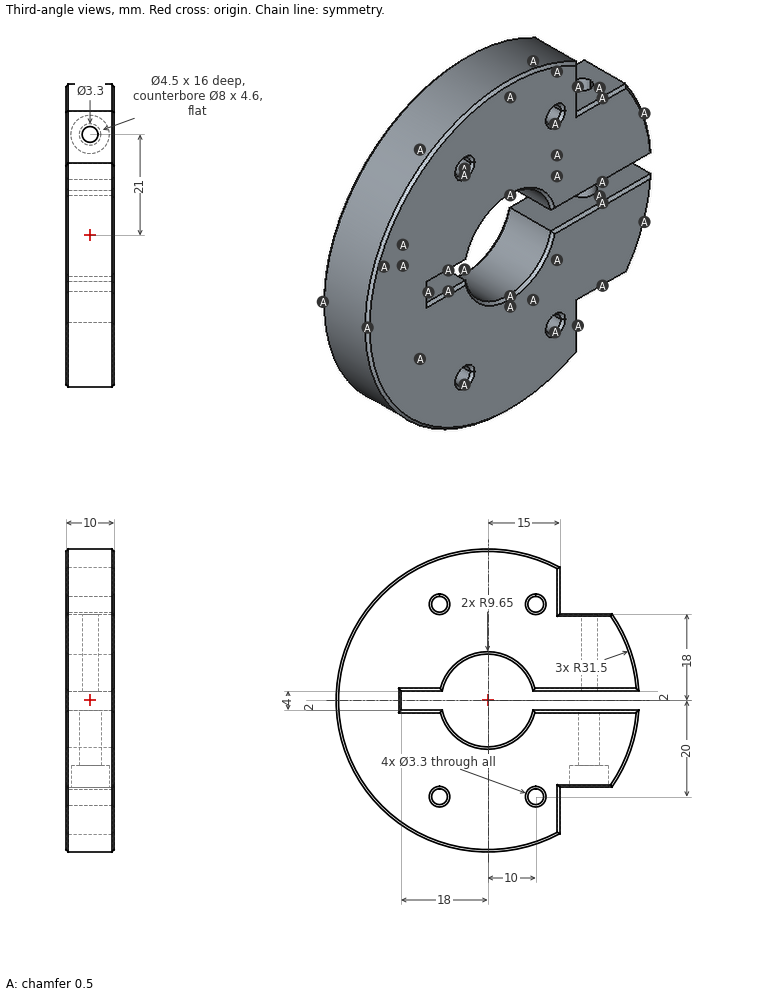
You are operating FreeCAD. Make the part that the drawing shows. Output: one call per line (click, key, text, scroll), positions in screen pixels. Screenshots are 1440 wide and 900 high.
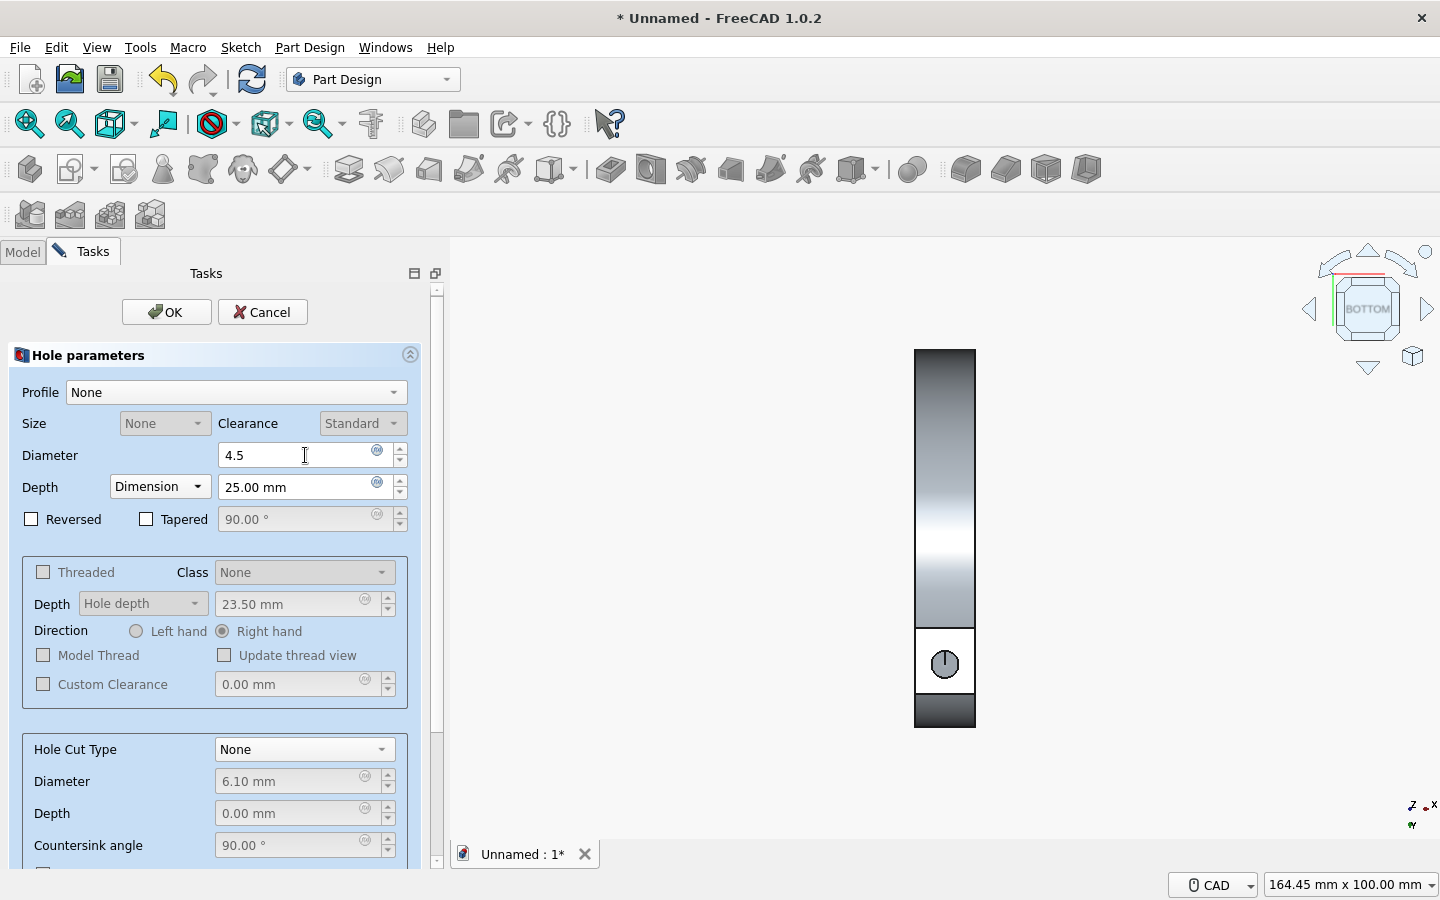
triple_click(305, 487)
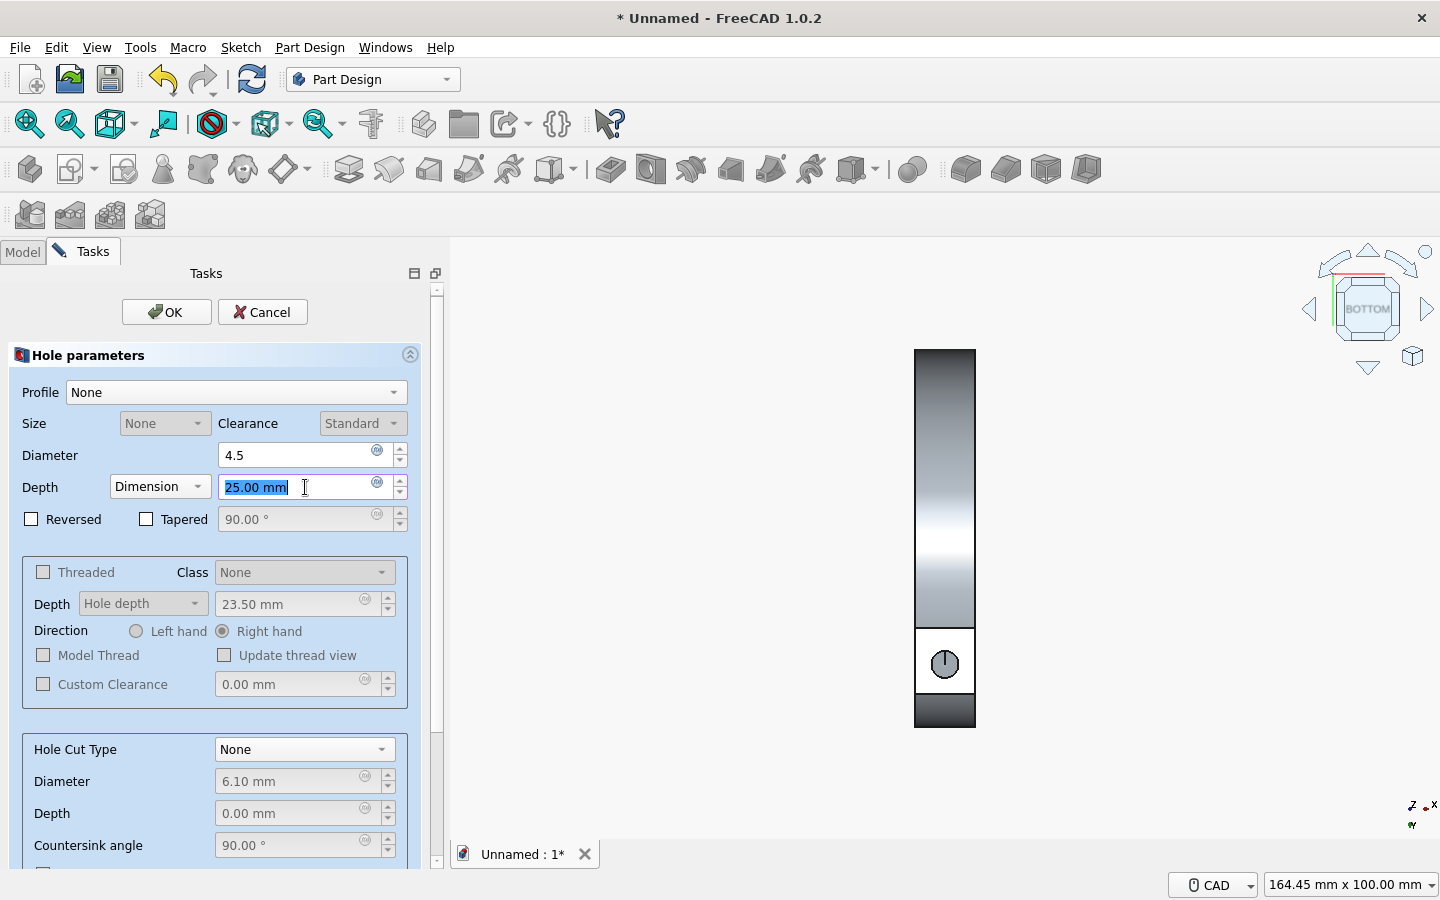
text(16)
key(Tab)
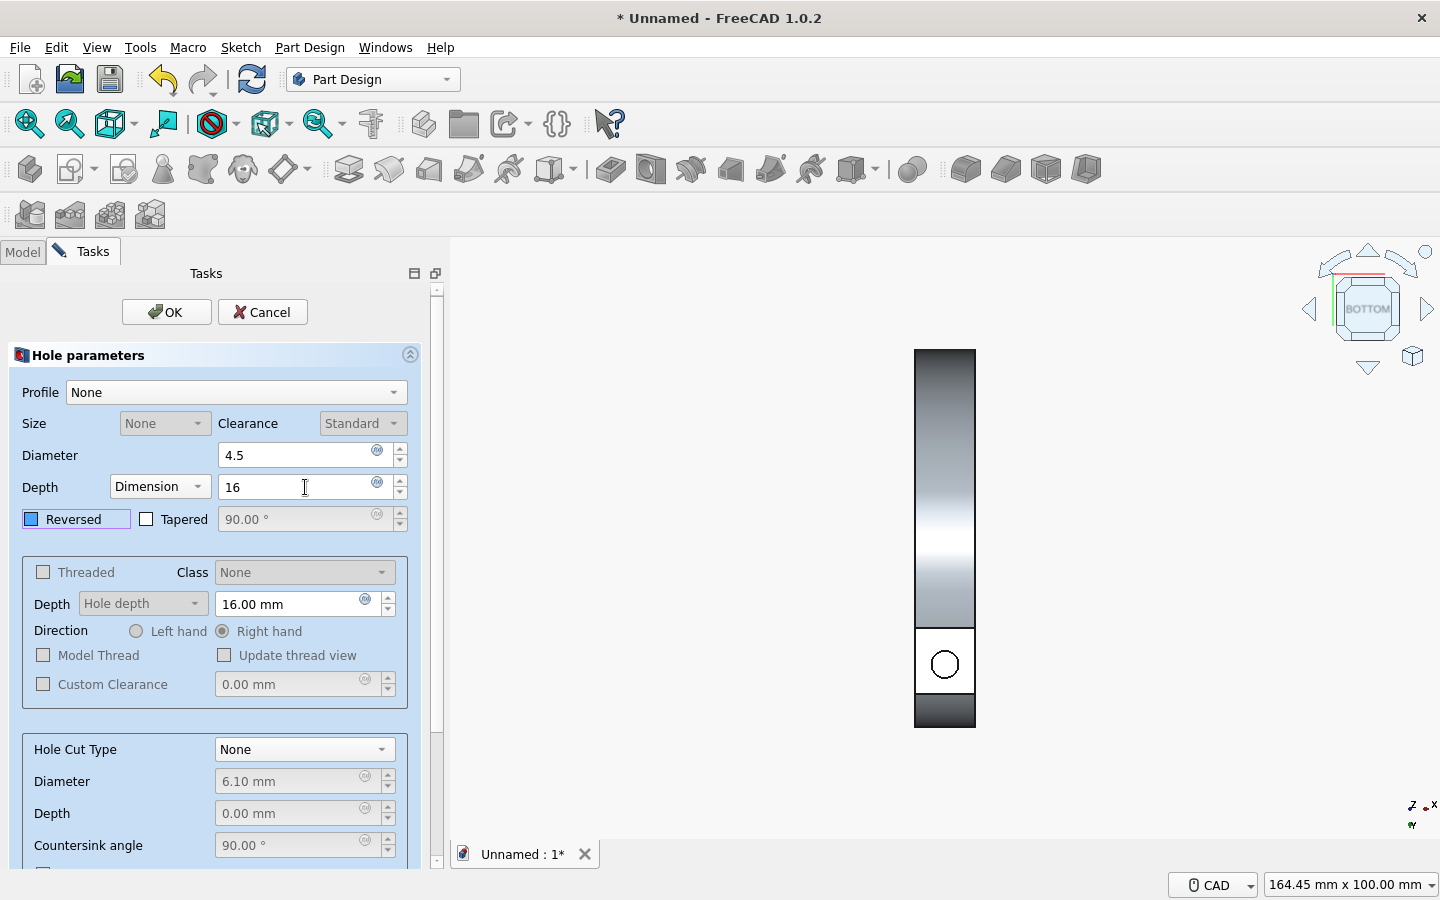
click(306, 750)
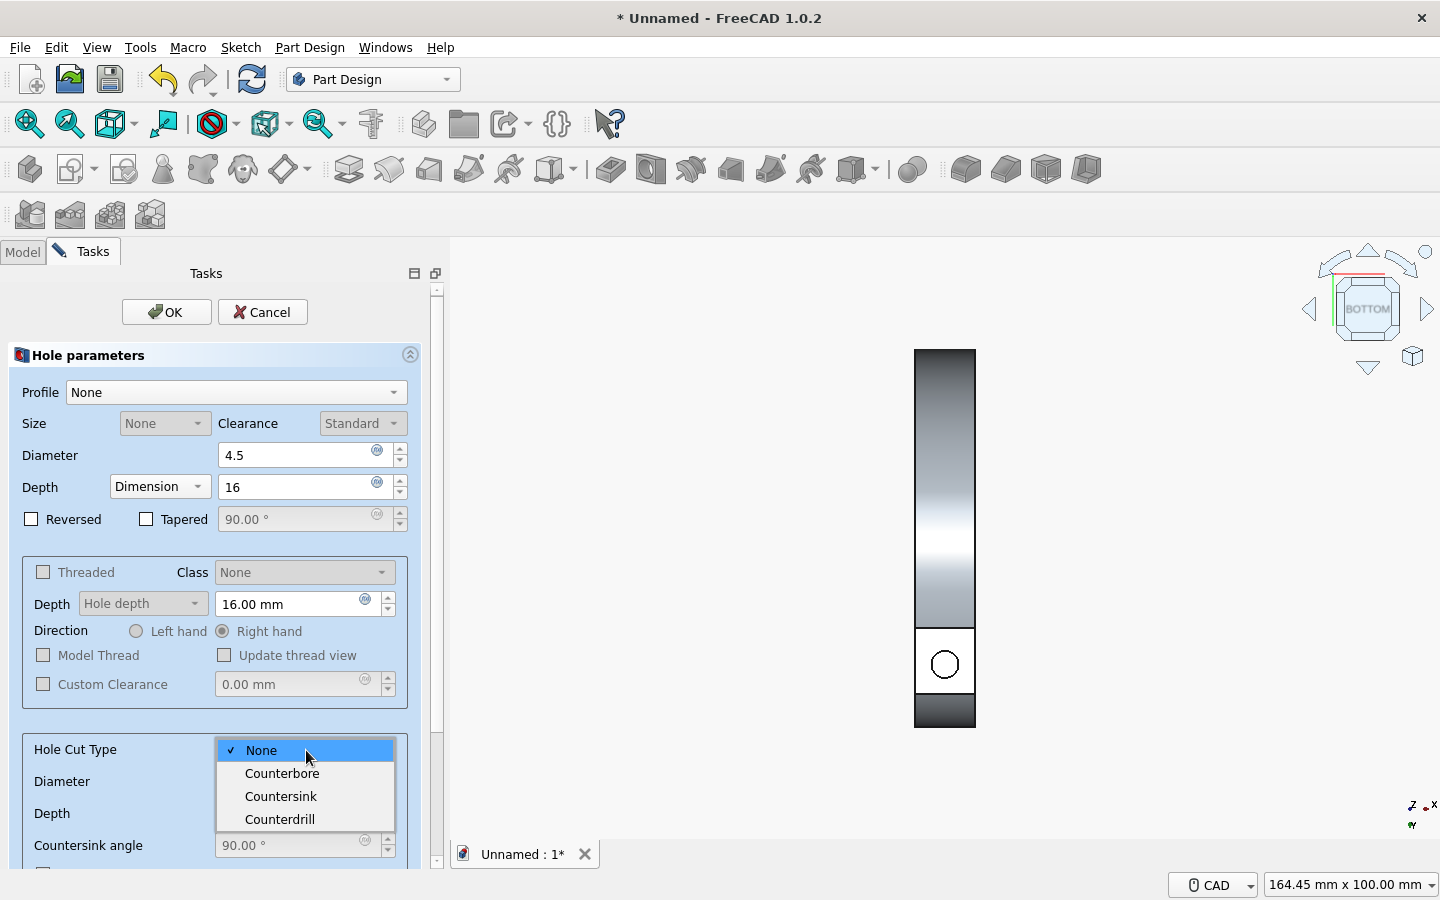
click(304, 774)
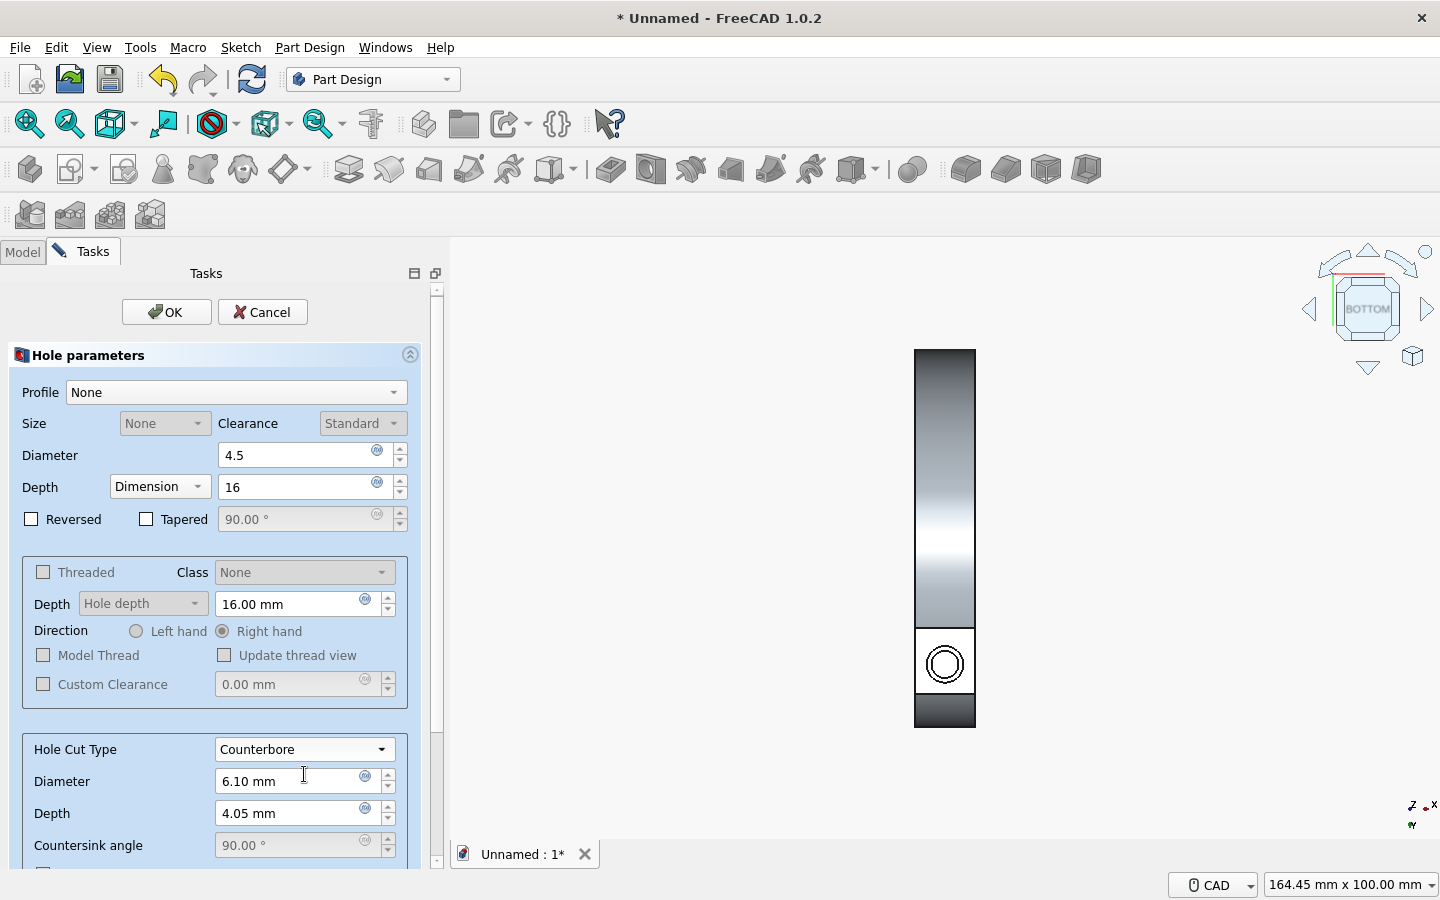
triple_click(298, 781)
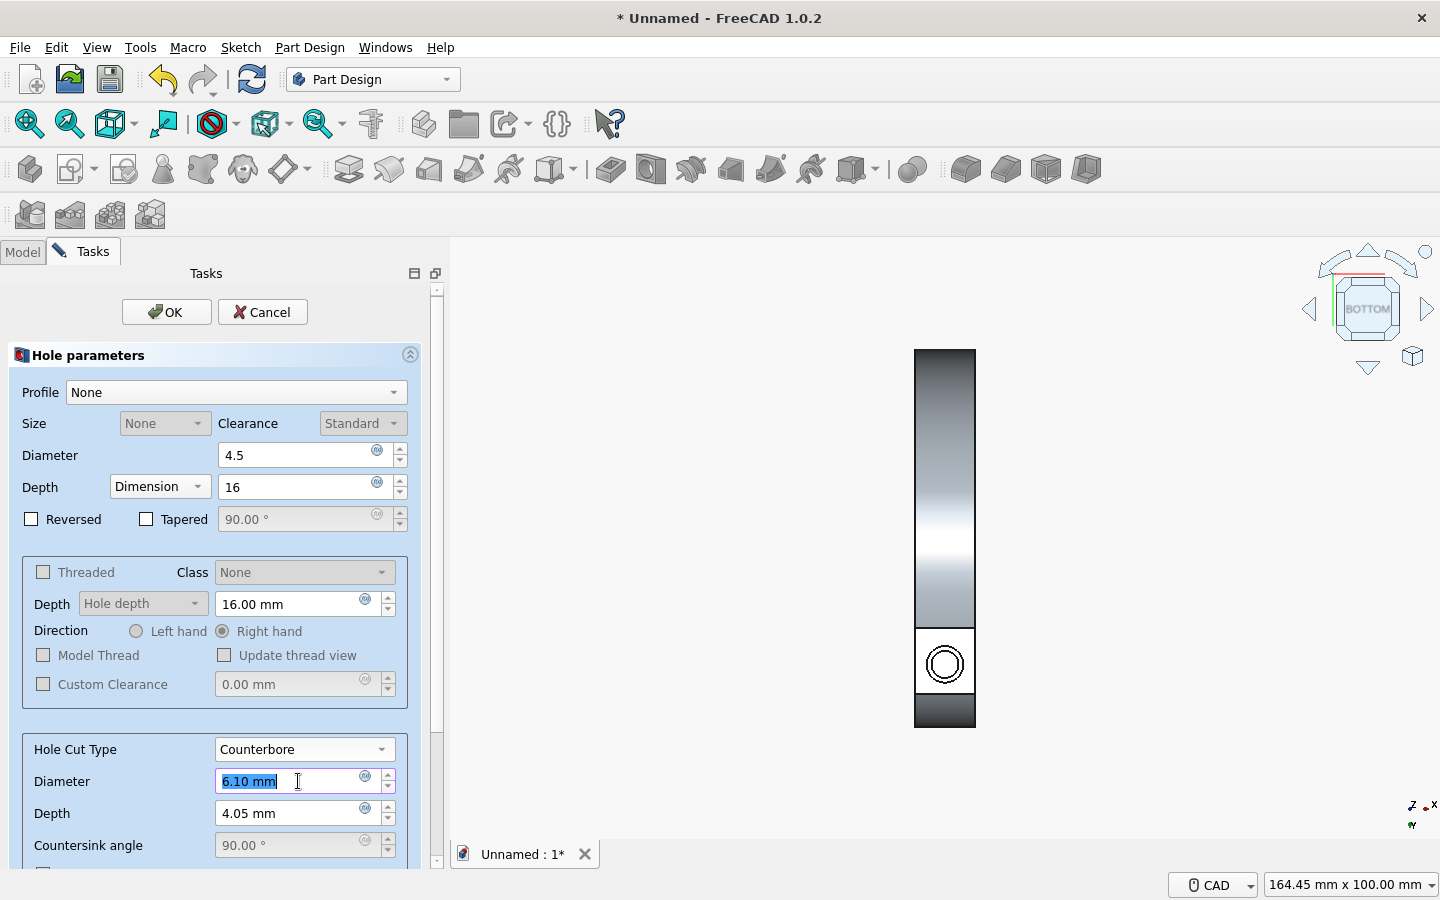
text(8)
key(Tab)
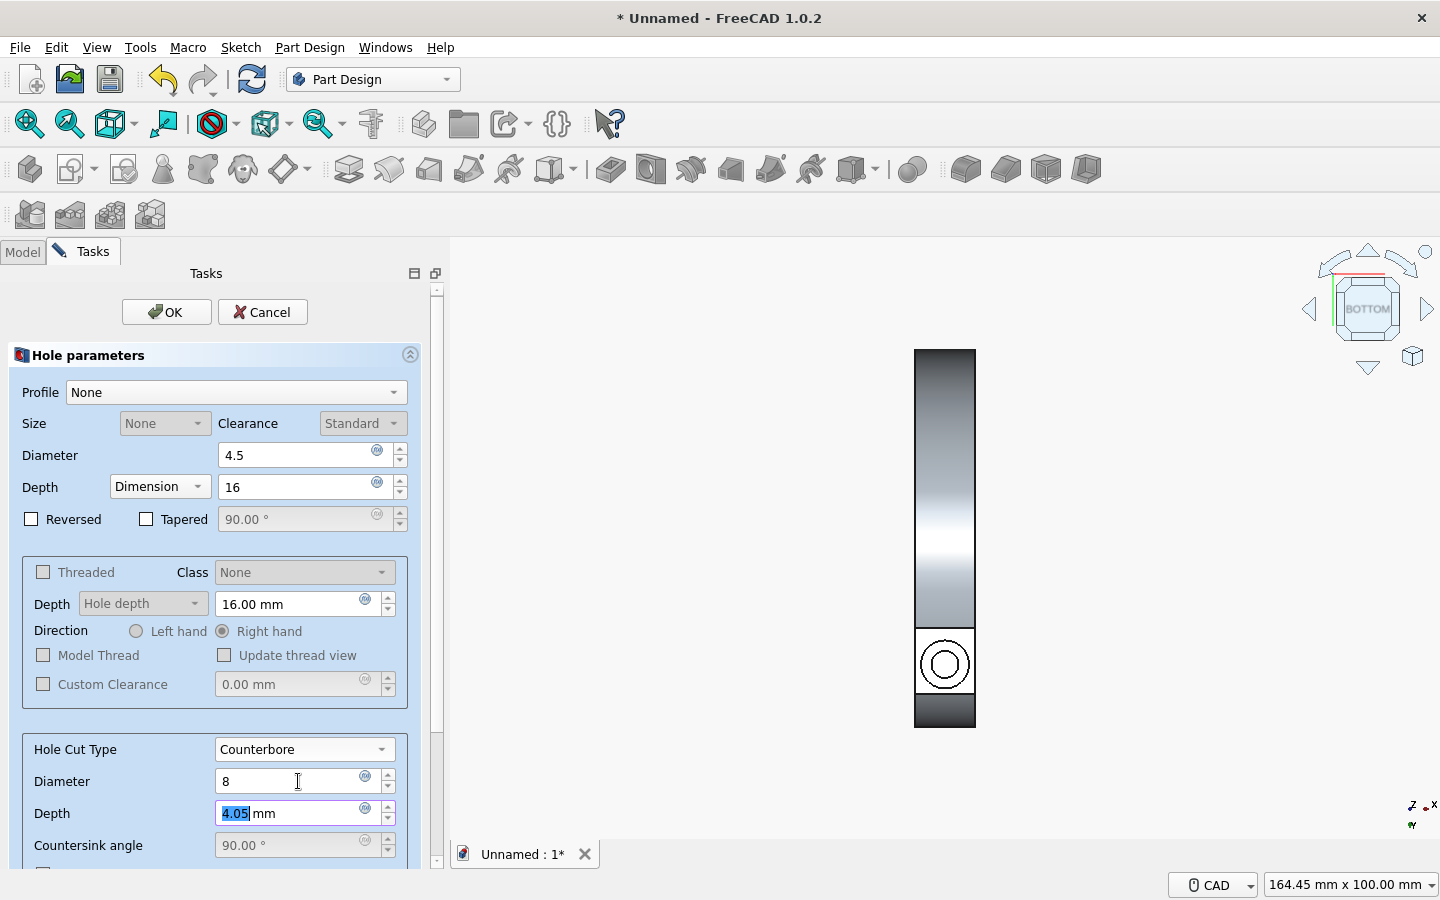
text(4.6)
key(Tab)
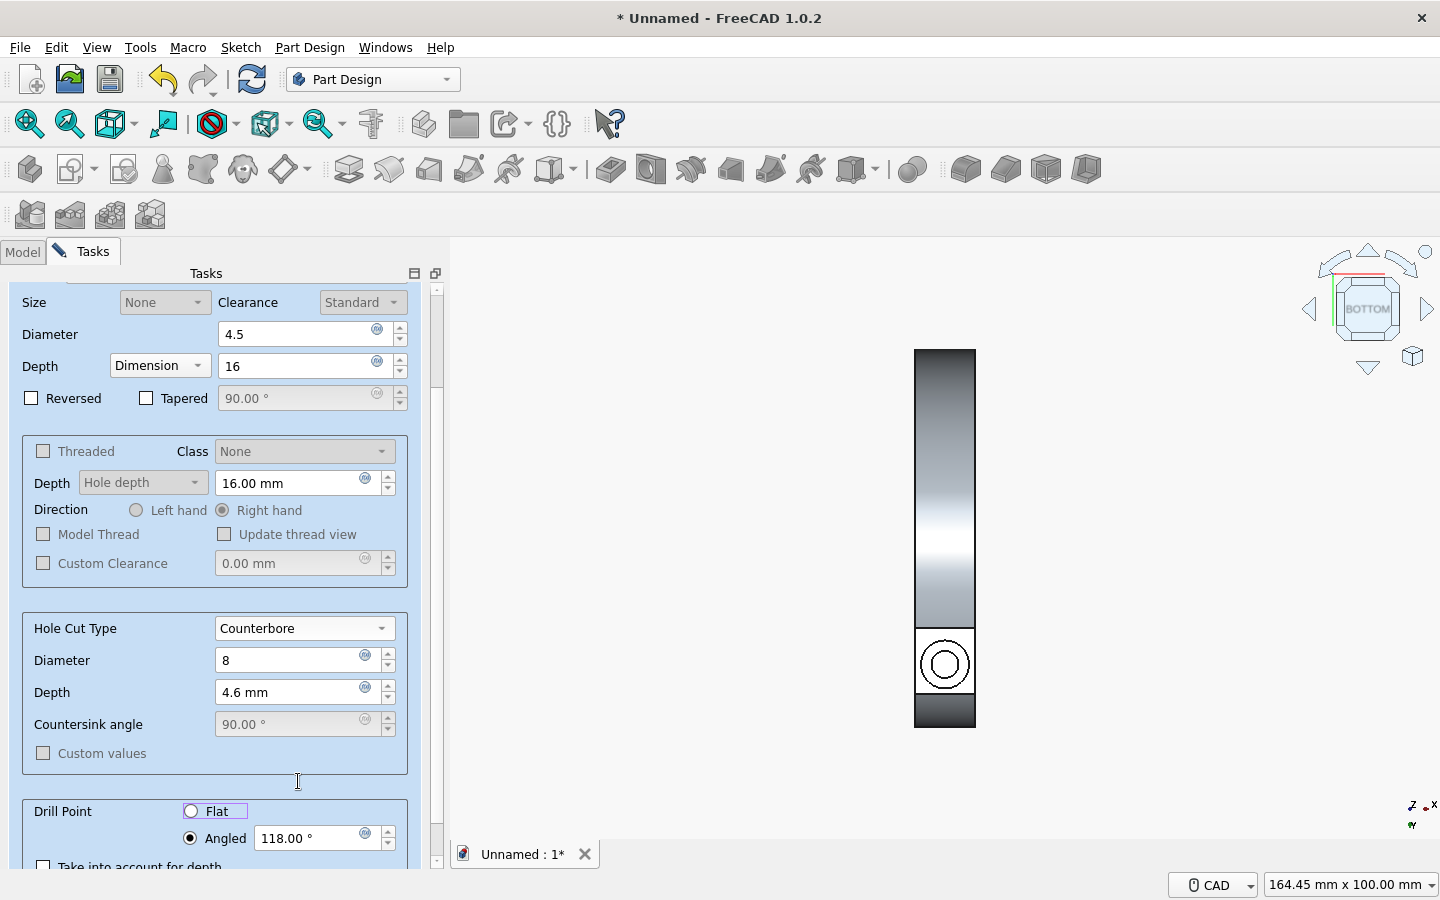
click(191, 811)